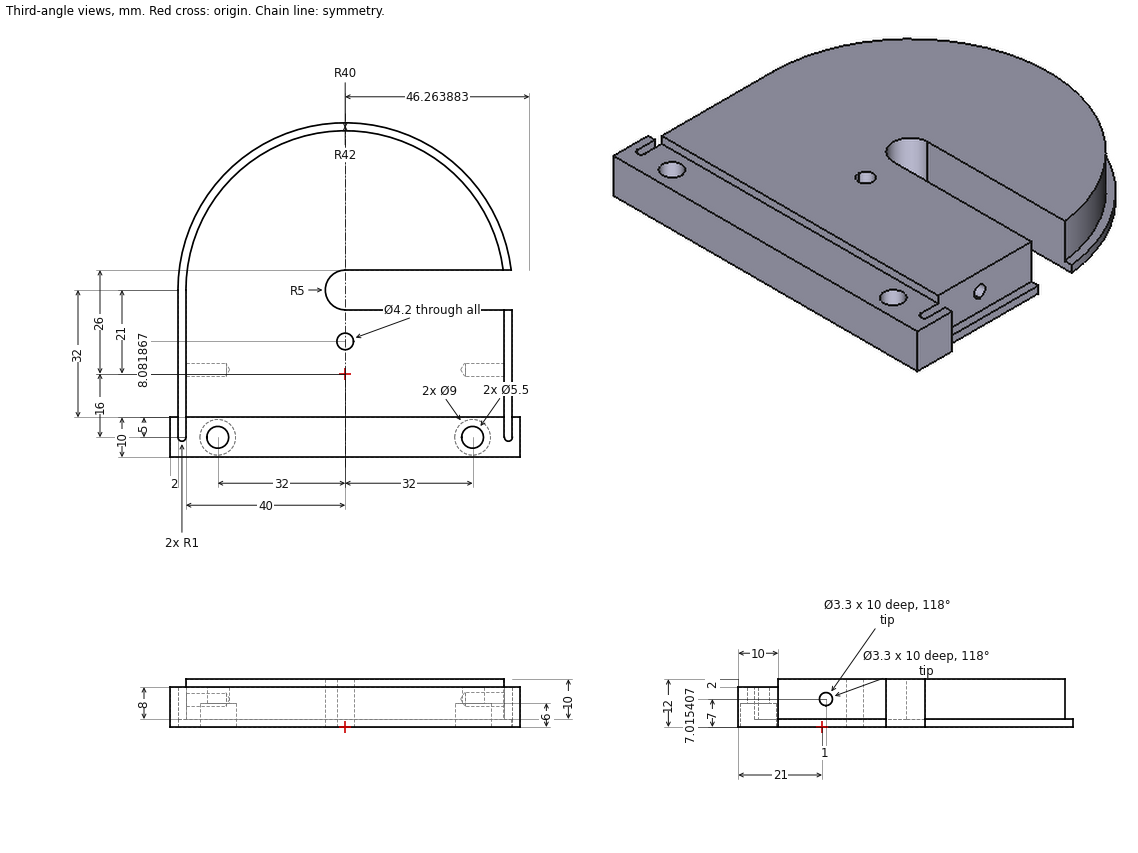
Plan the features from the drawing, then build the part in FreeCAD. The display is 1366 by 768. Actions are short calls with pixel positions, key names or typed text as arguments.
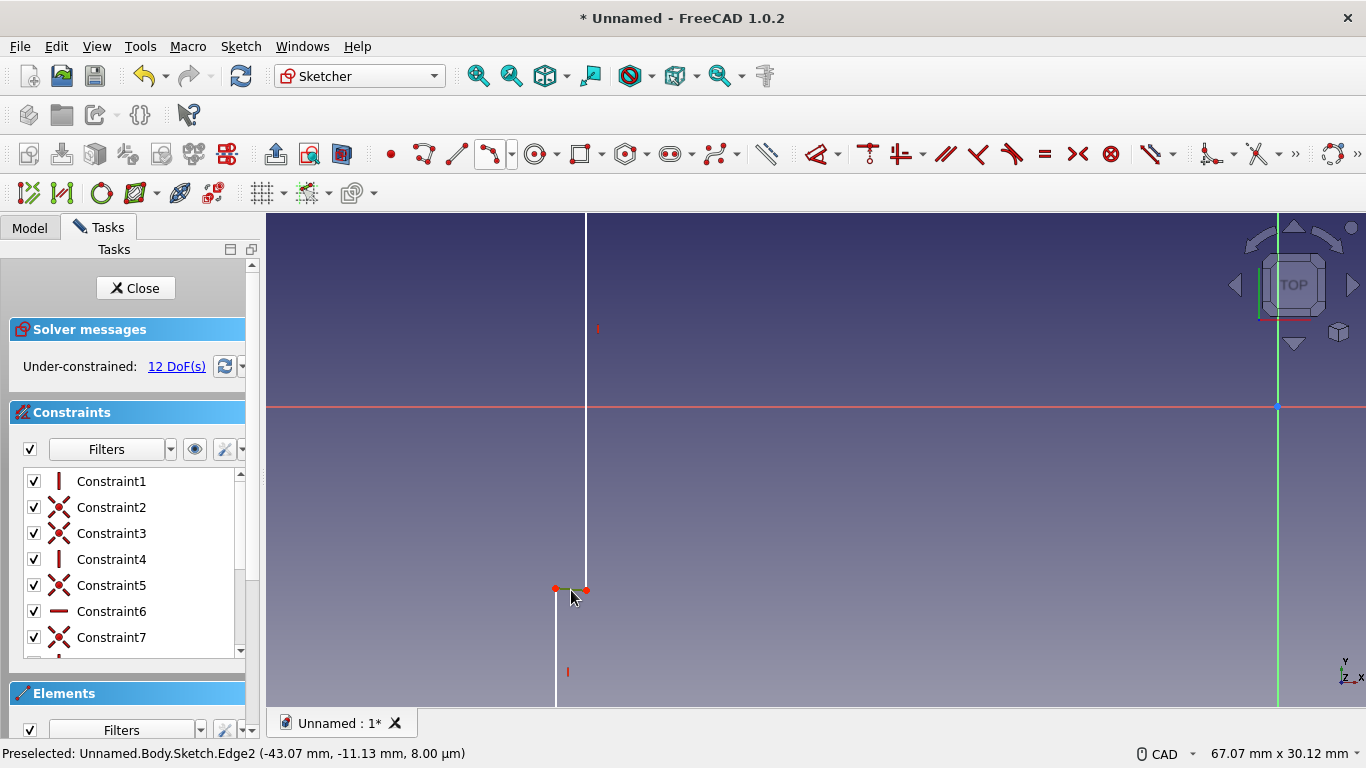
key(h)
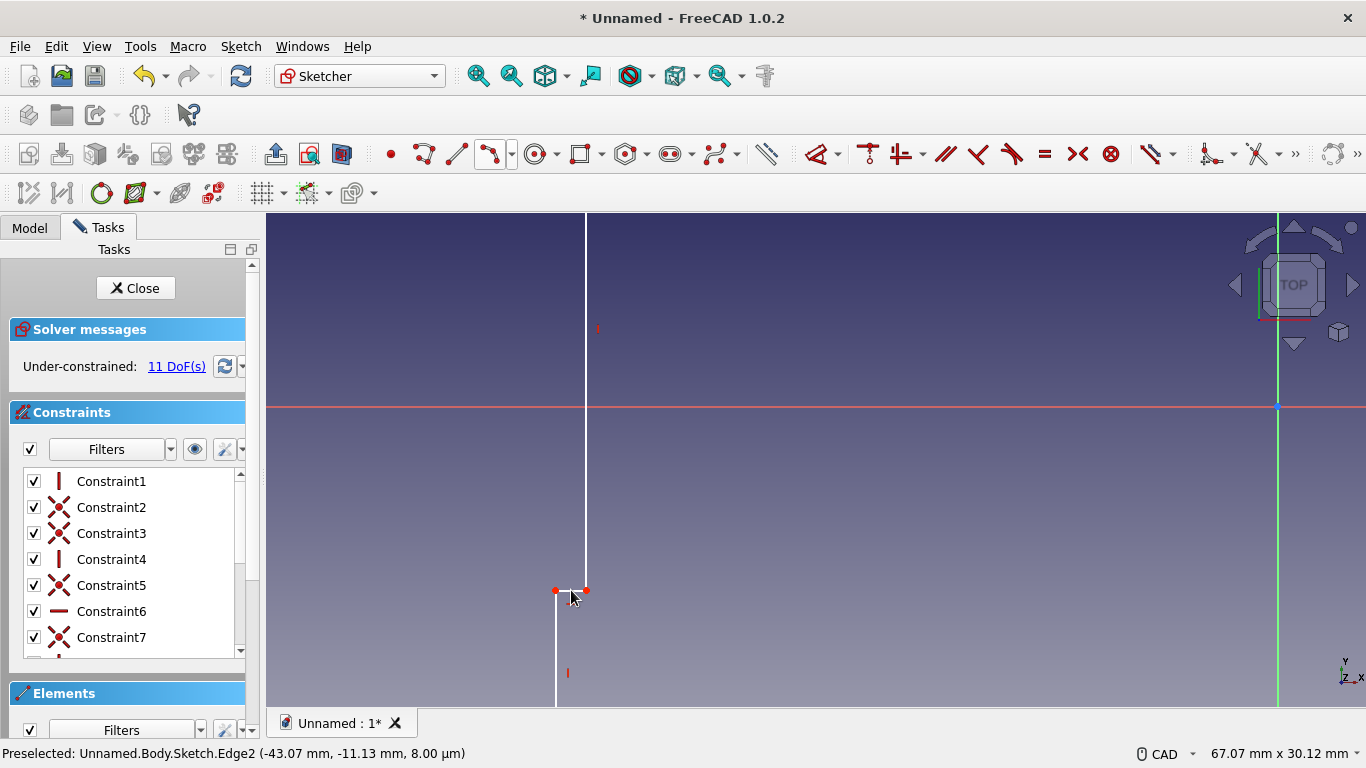
scroll(574, 590, down, 7)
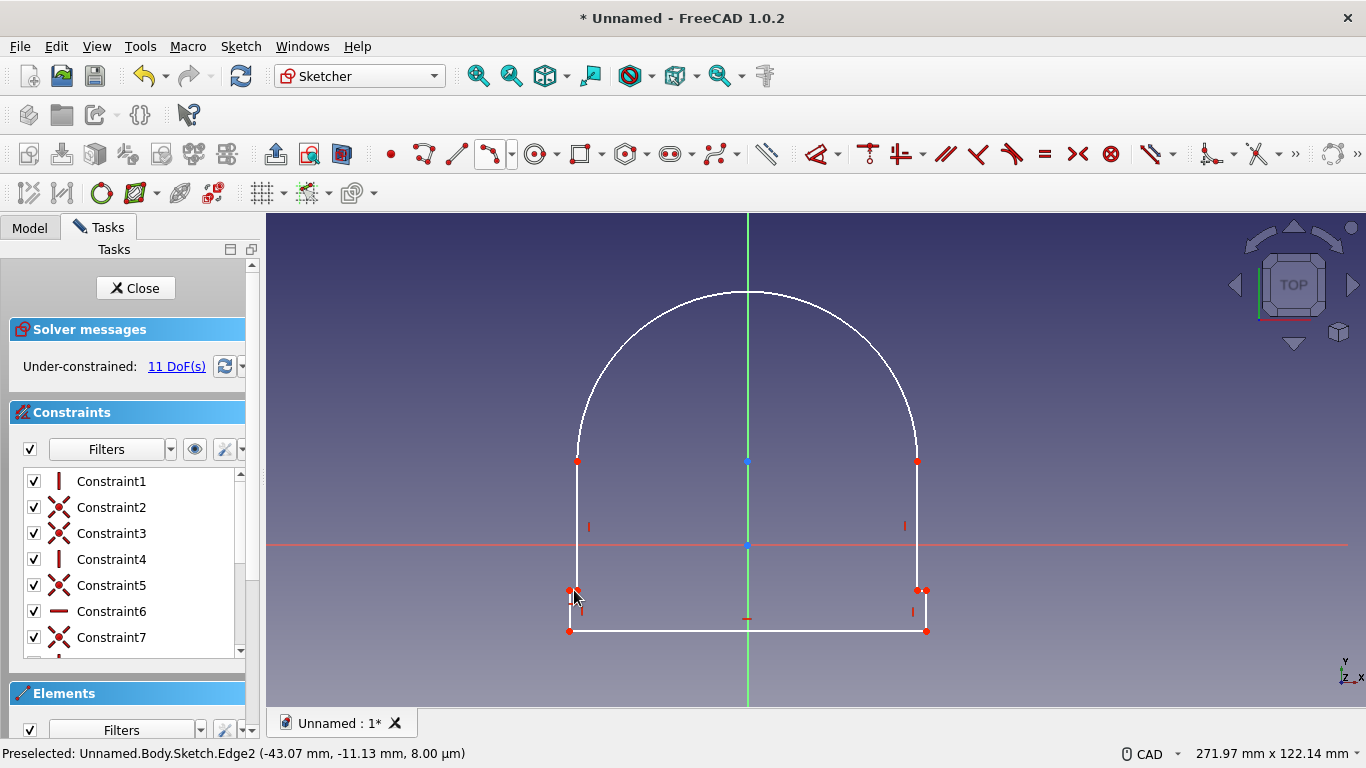
scroll(923, 591, up, 9)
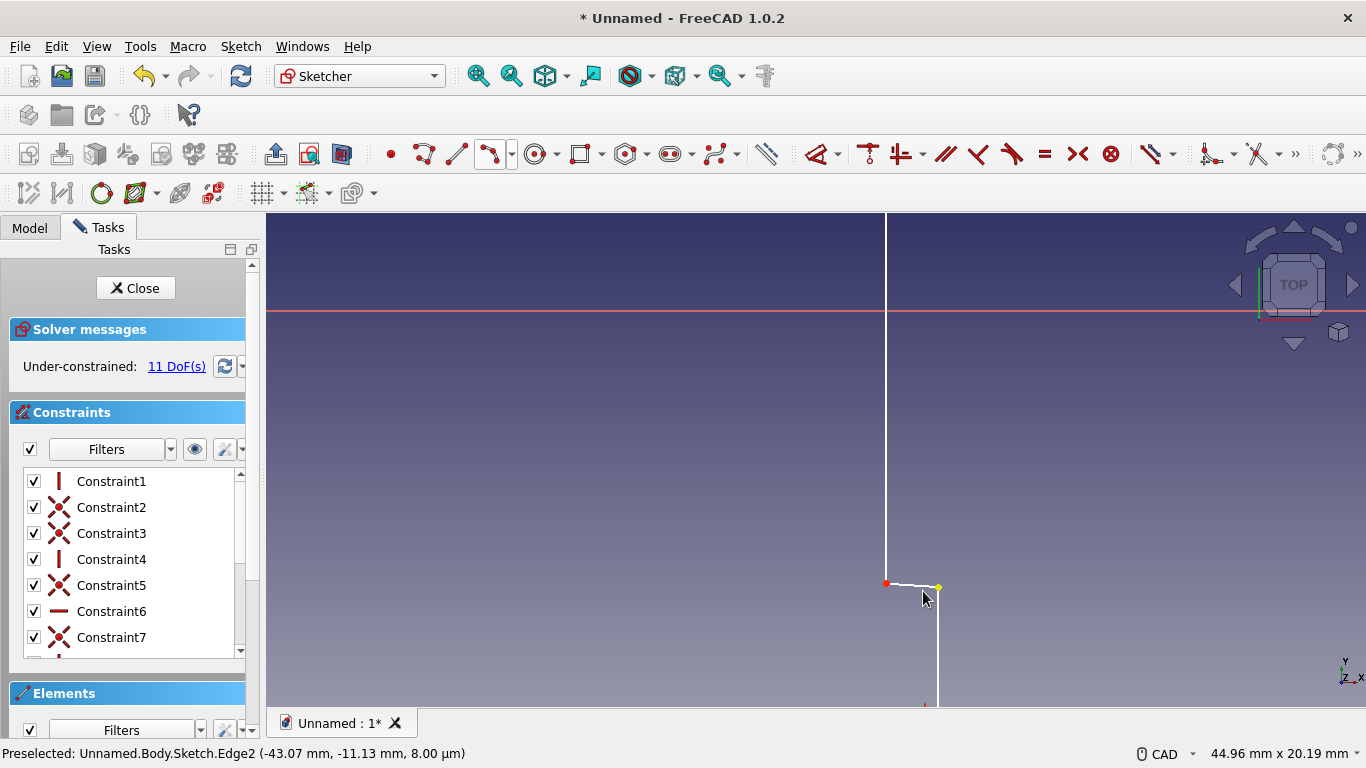
click(923, 586)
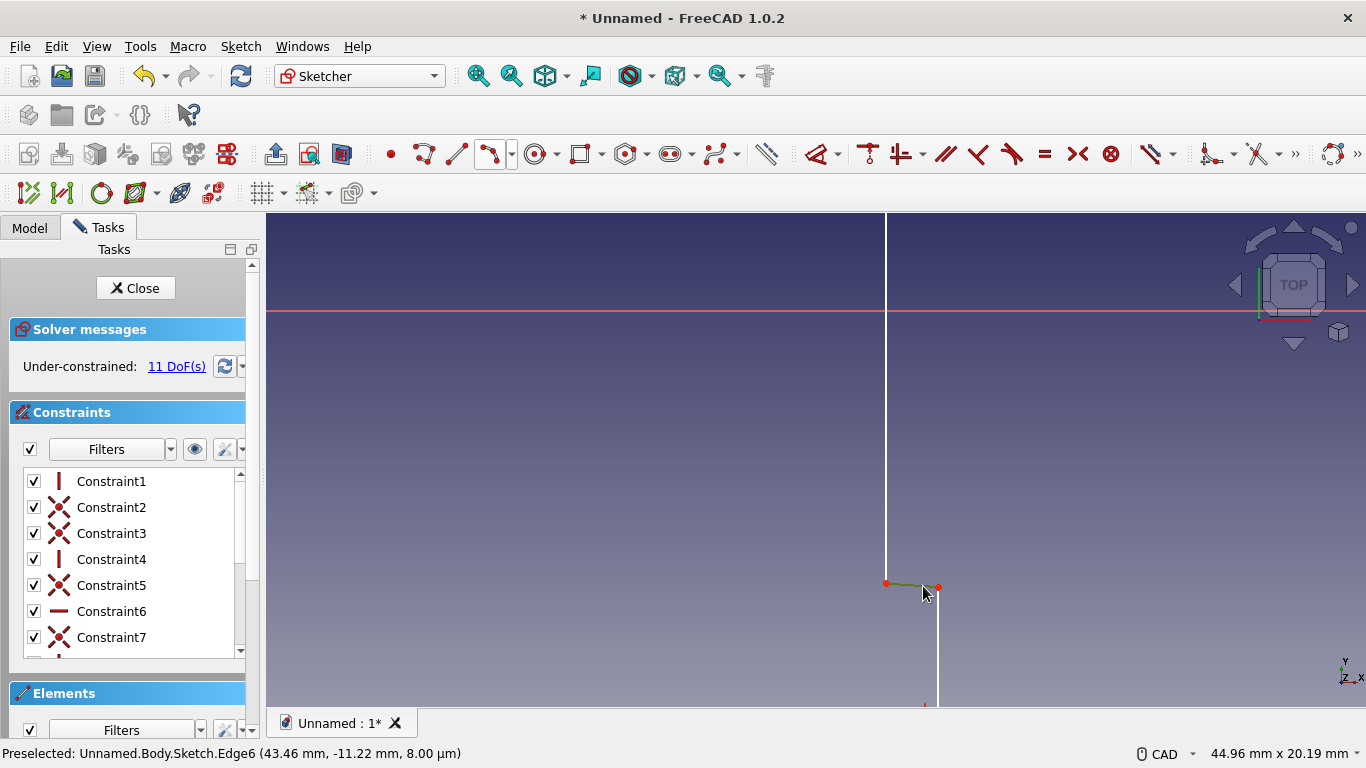
key(h)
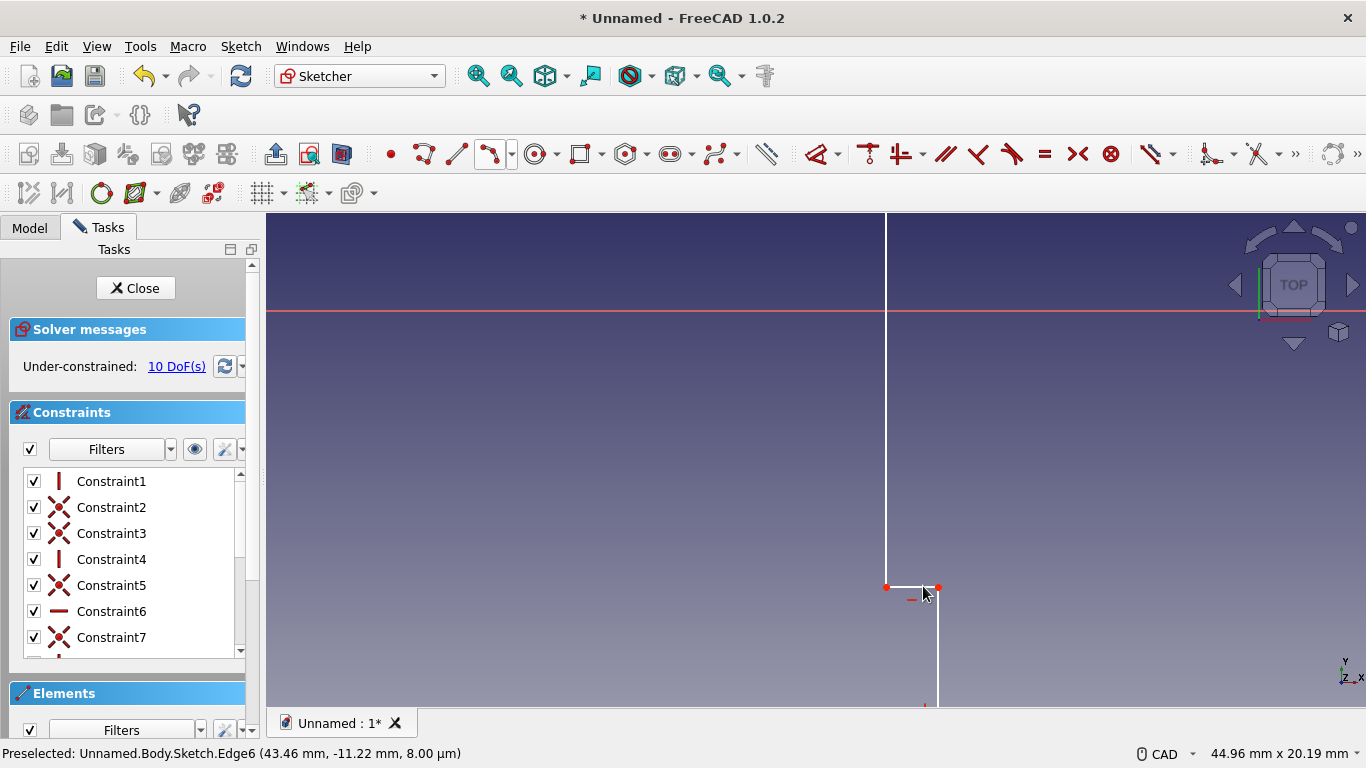
scroll(923, 591, down, 9)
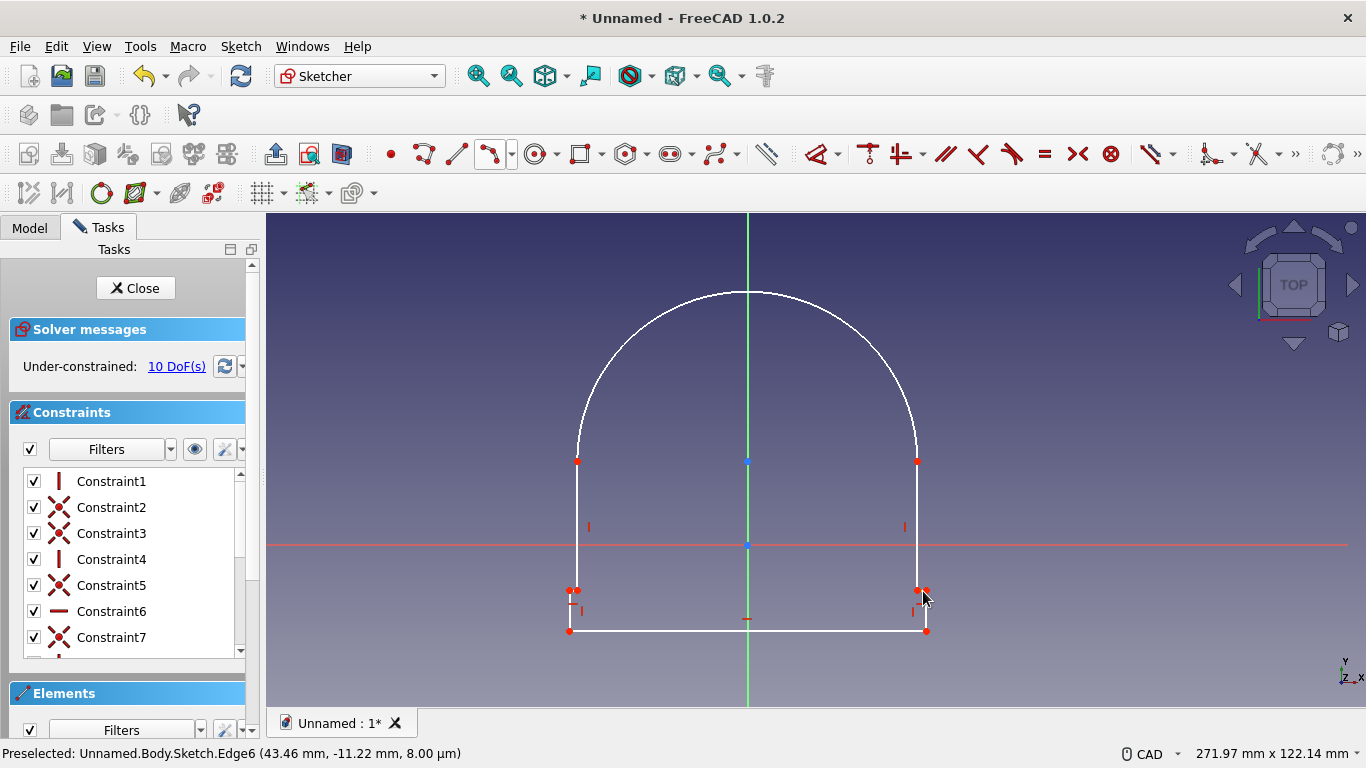
click(747, 462)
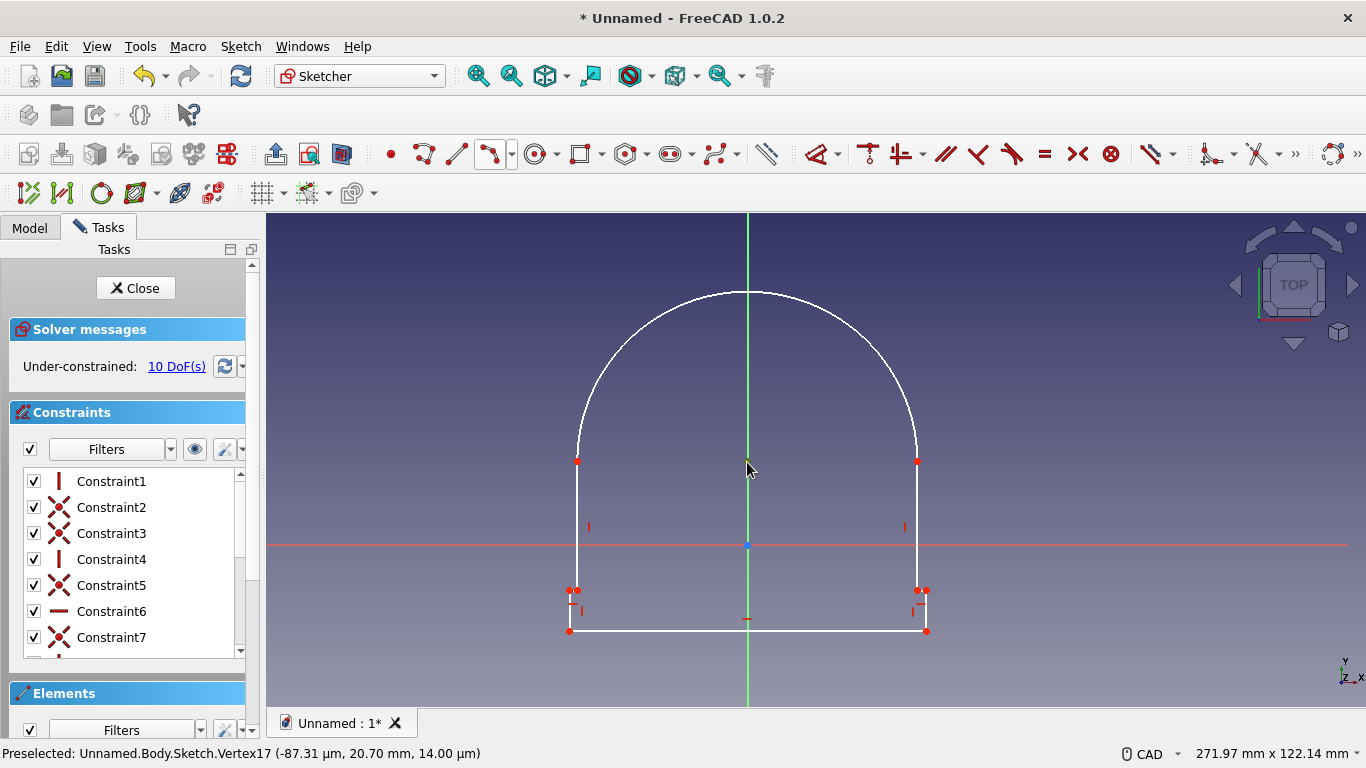
click(748, 585)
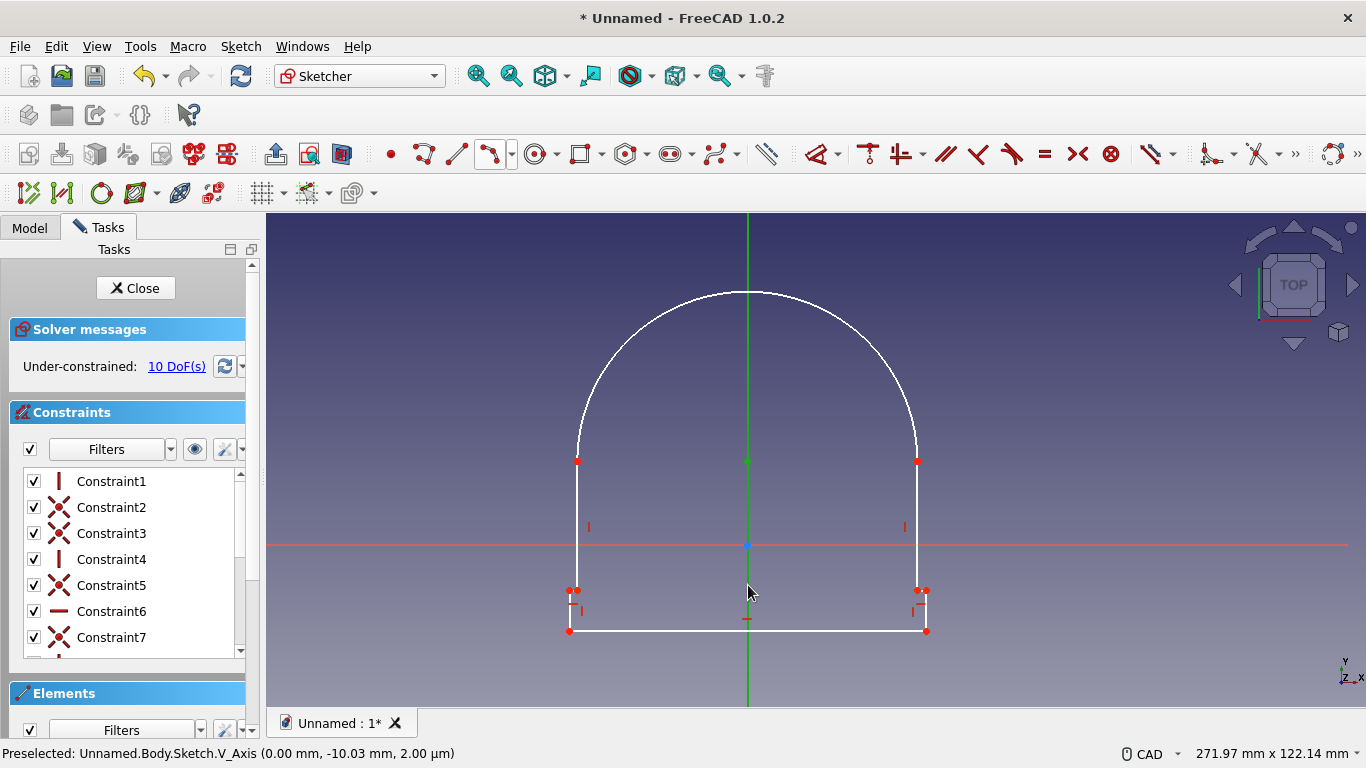
click(868, 154)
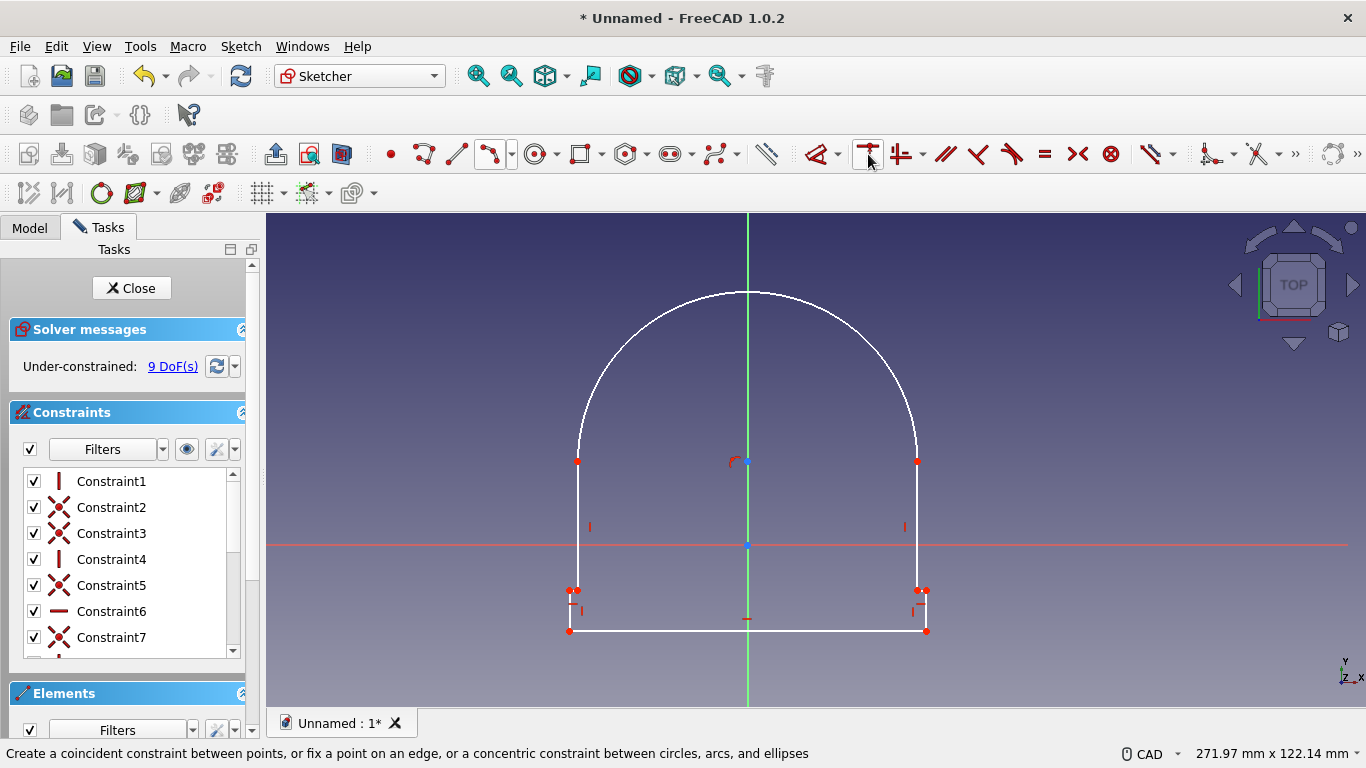
scroll(570, 591, up, 2)